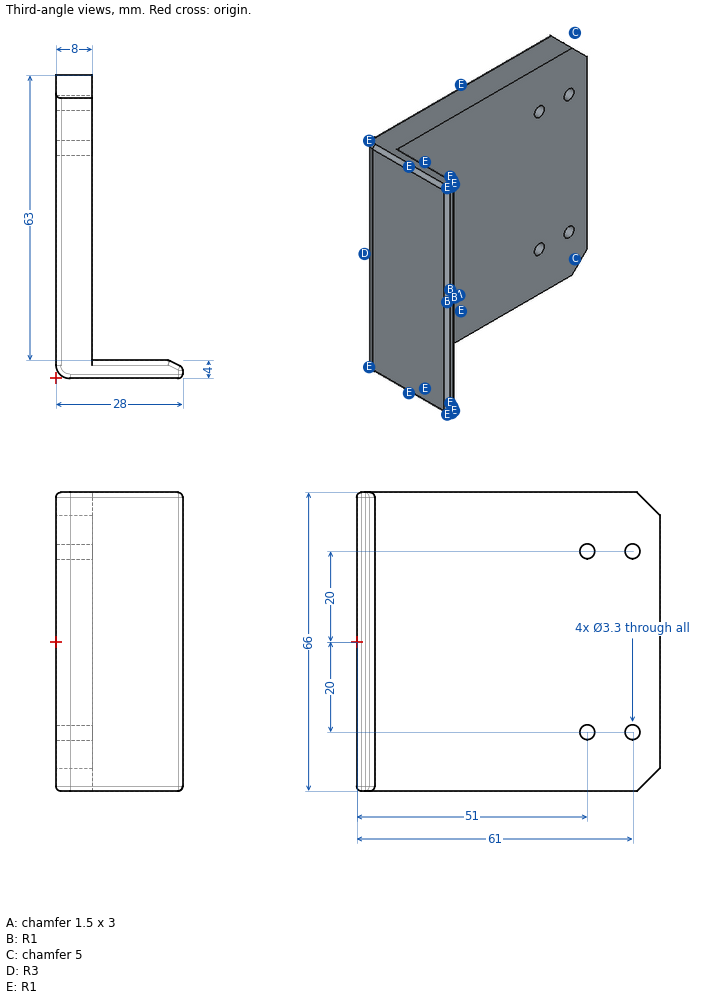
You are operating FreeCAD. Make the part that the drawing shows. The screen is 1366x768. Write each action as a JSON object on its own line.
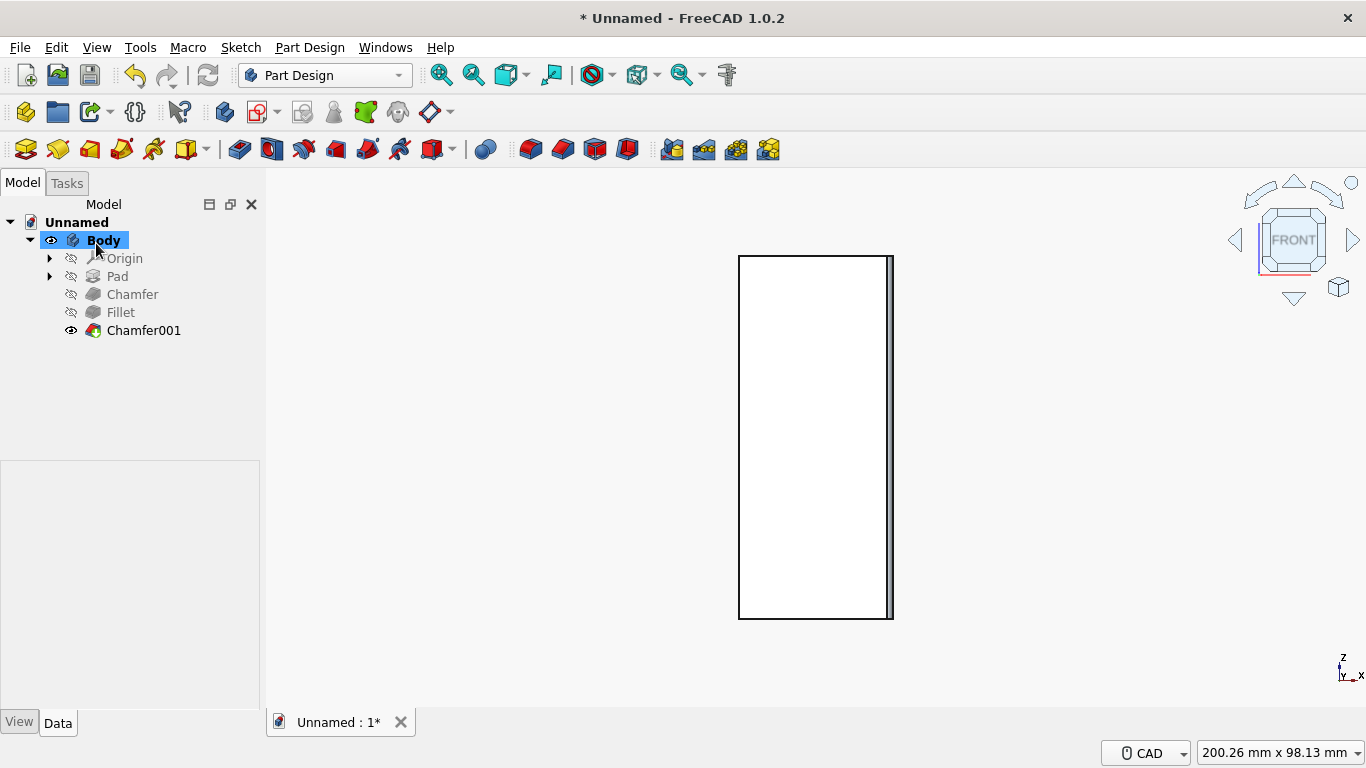
{"action": "left_click", "coordinate": [739, 437]}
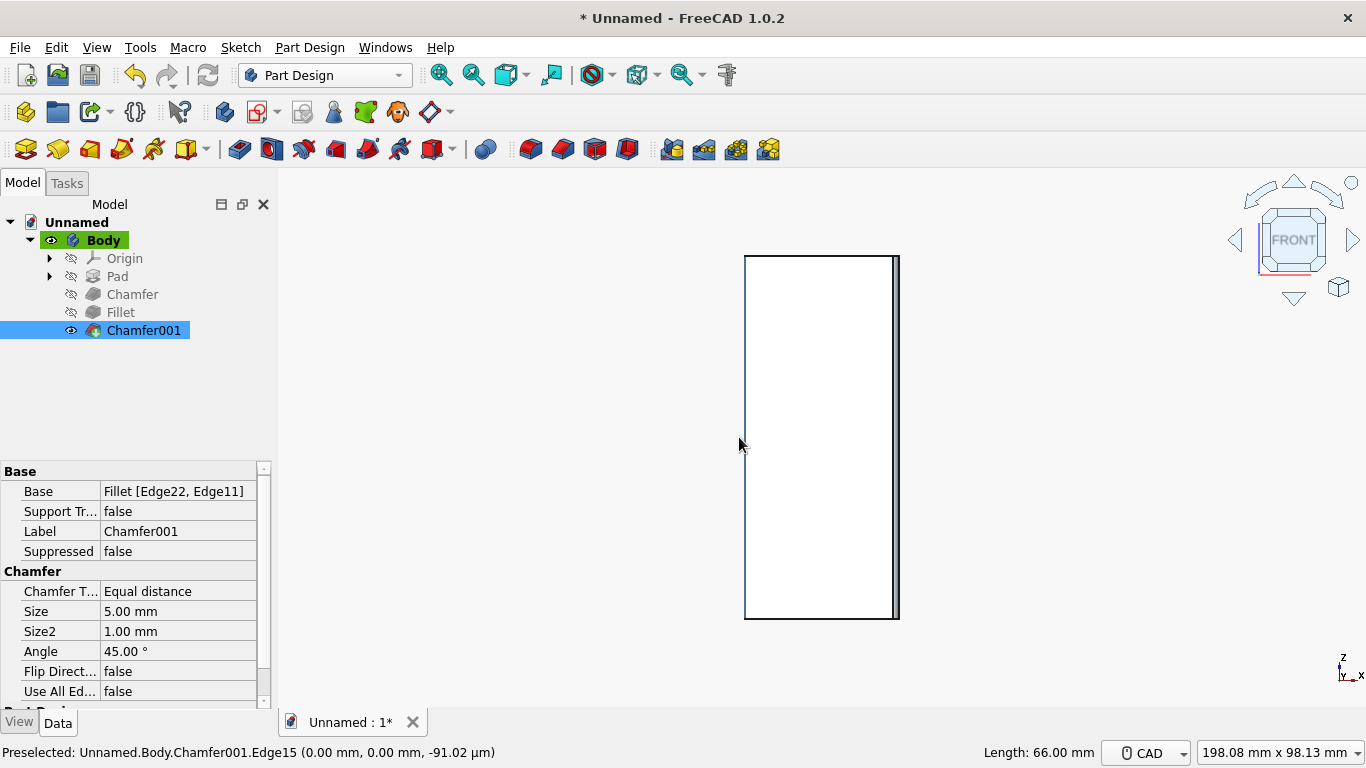
{"action": "left_click", "coordinate": [532, 150]}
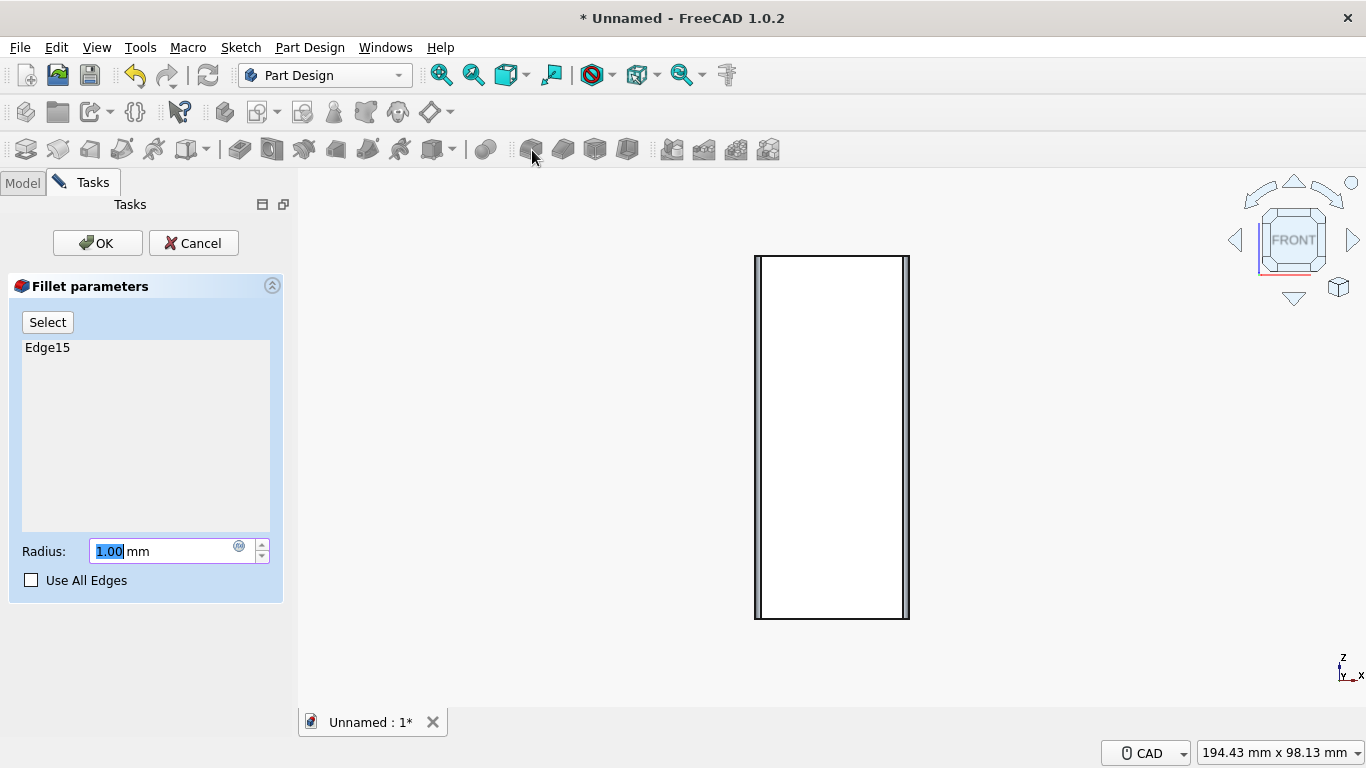
{"action": "type", "text": "3"}
{"action": "key", "text": "Tab"}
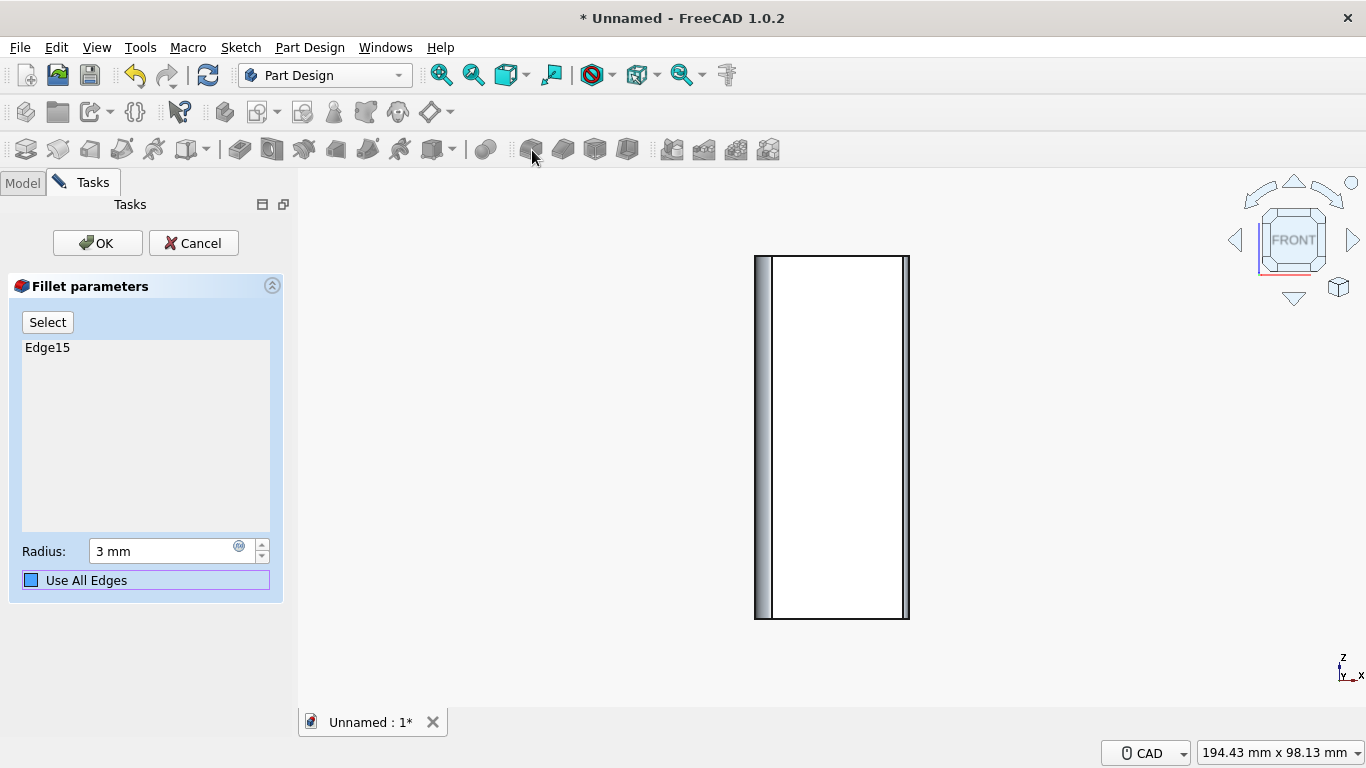
{"action": "left_click", "coordinate": [98, 243]}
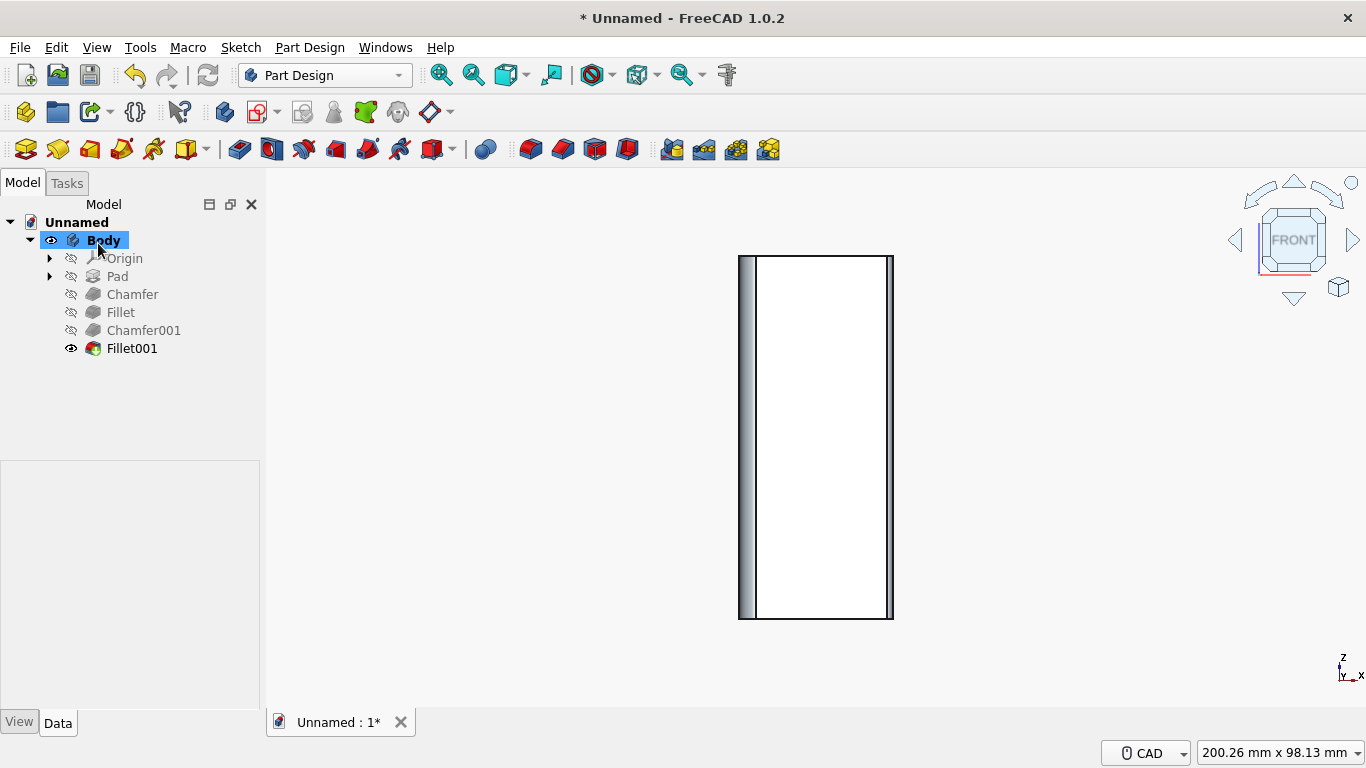
{"action": "left_click", "coordinate": [821, 618]}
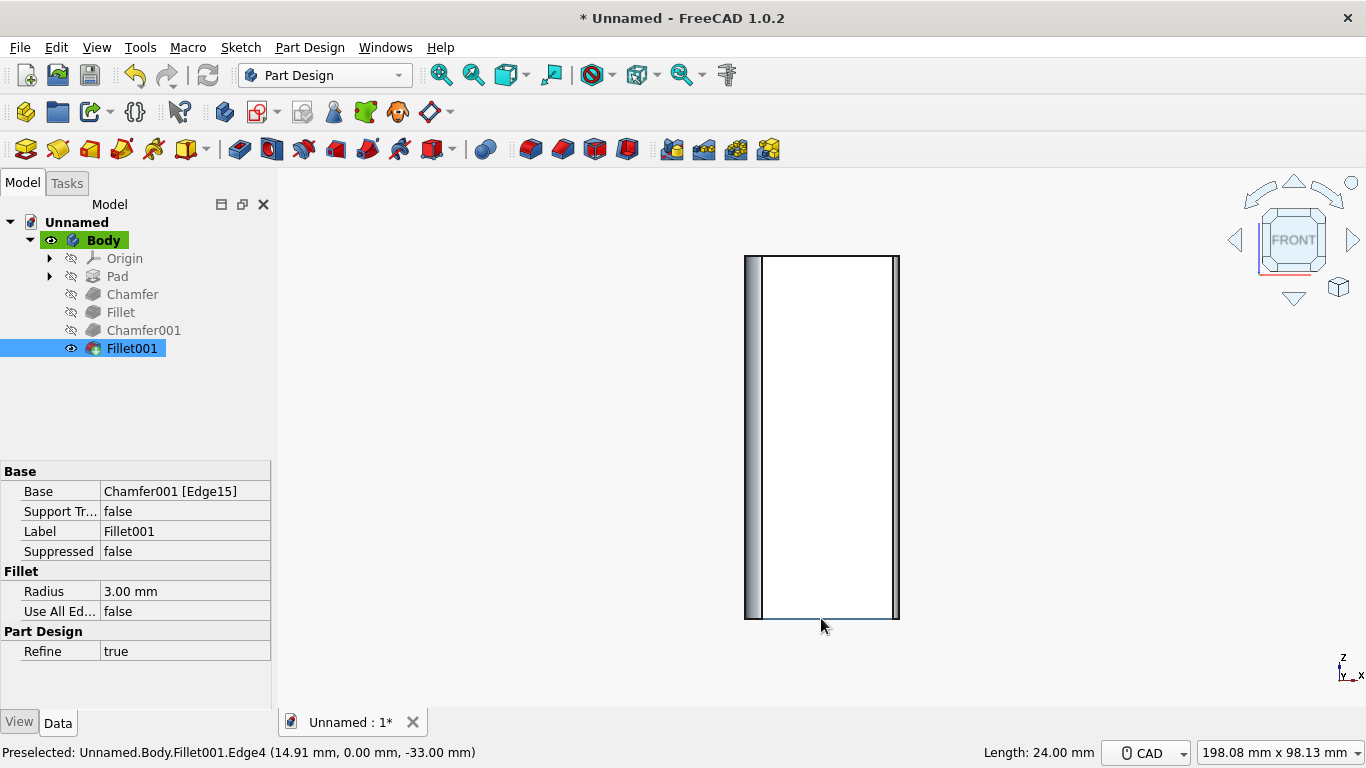
{"action": "left_click", "coordinate": [827, 255], "text": "ctrl"}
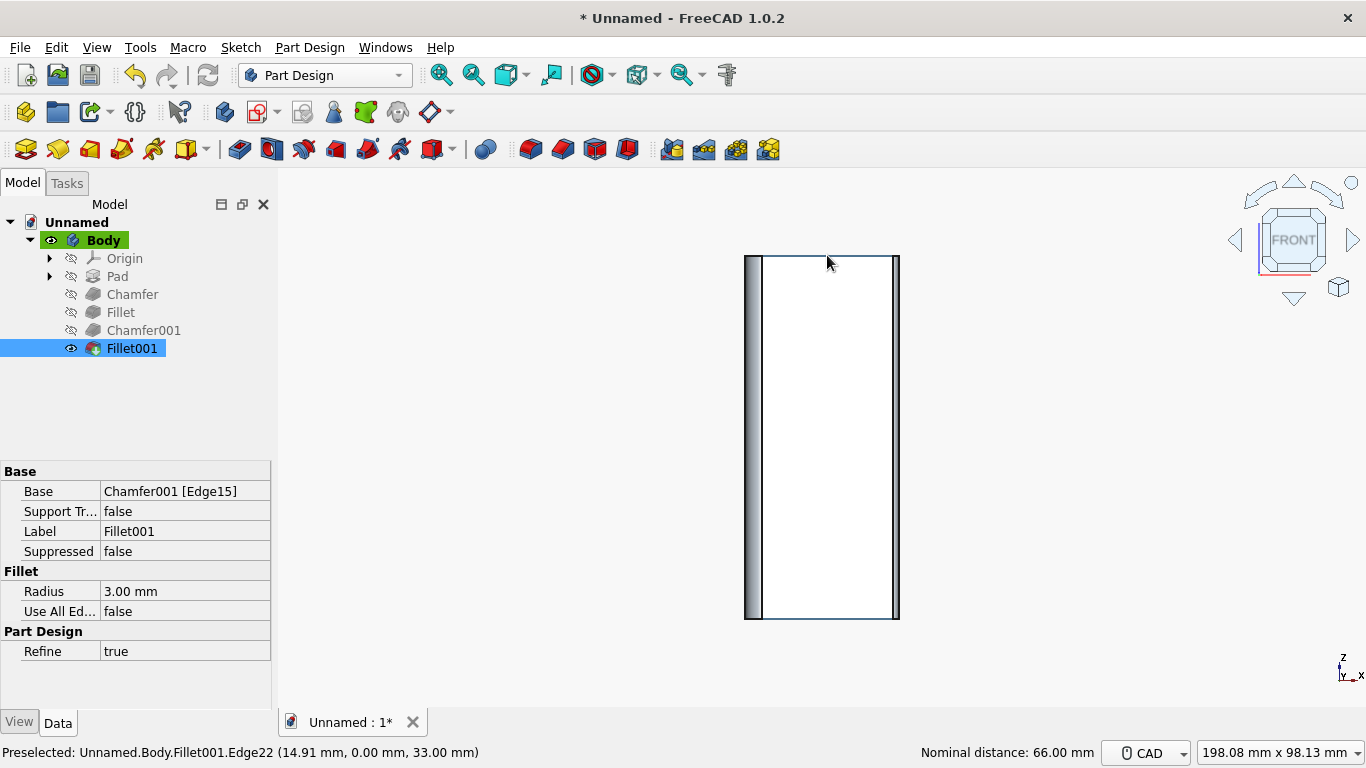
{"action": "left_click", "coordinate": [750, 618], "text": "ctrl"}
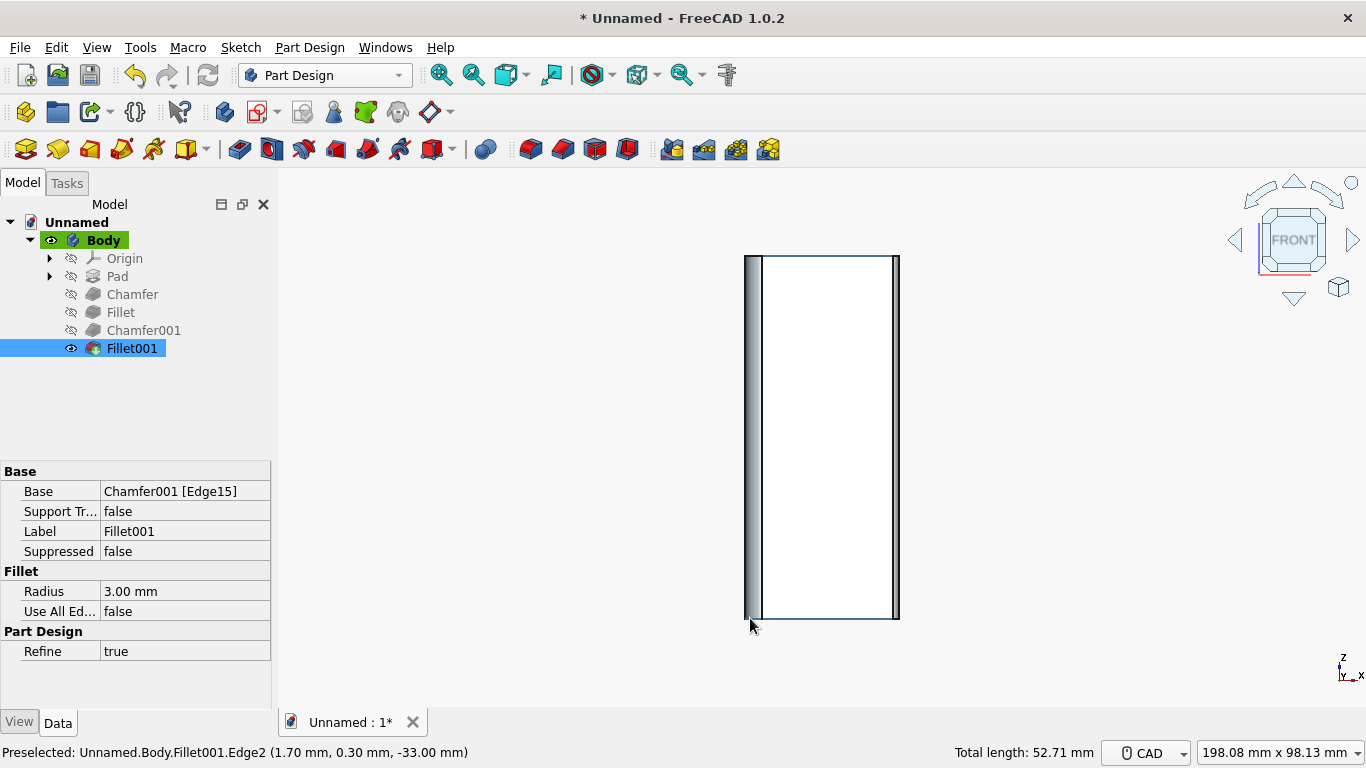
{"action": "left_click", "coordinate": [750, 255], "text": "ctrl"}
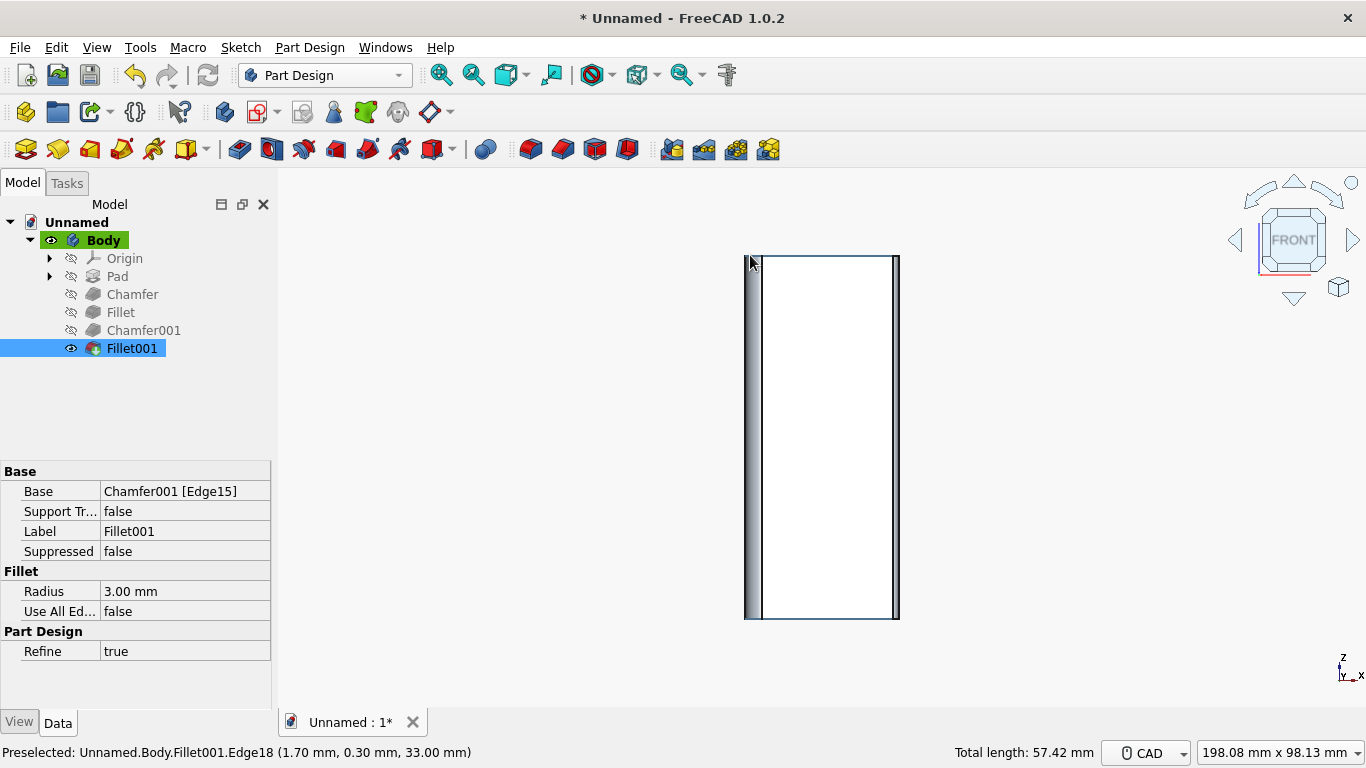
{"action": "scroll", "coordinate": [899, 618], "scroll_direction": "up", "scroll_amount": 11}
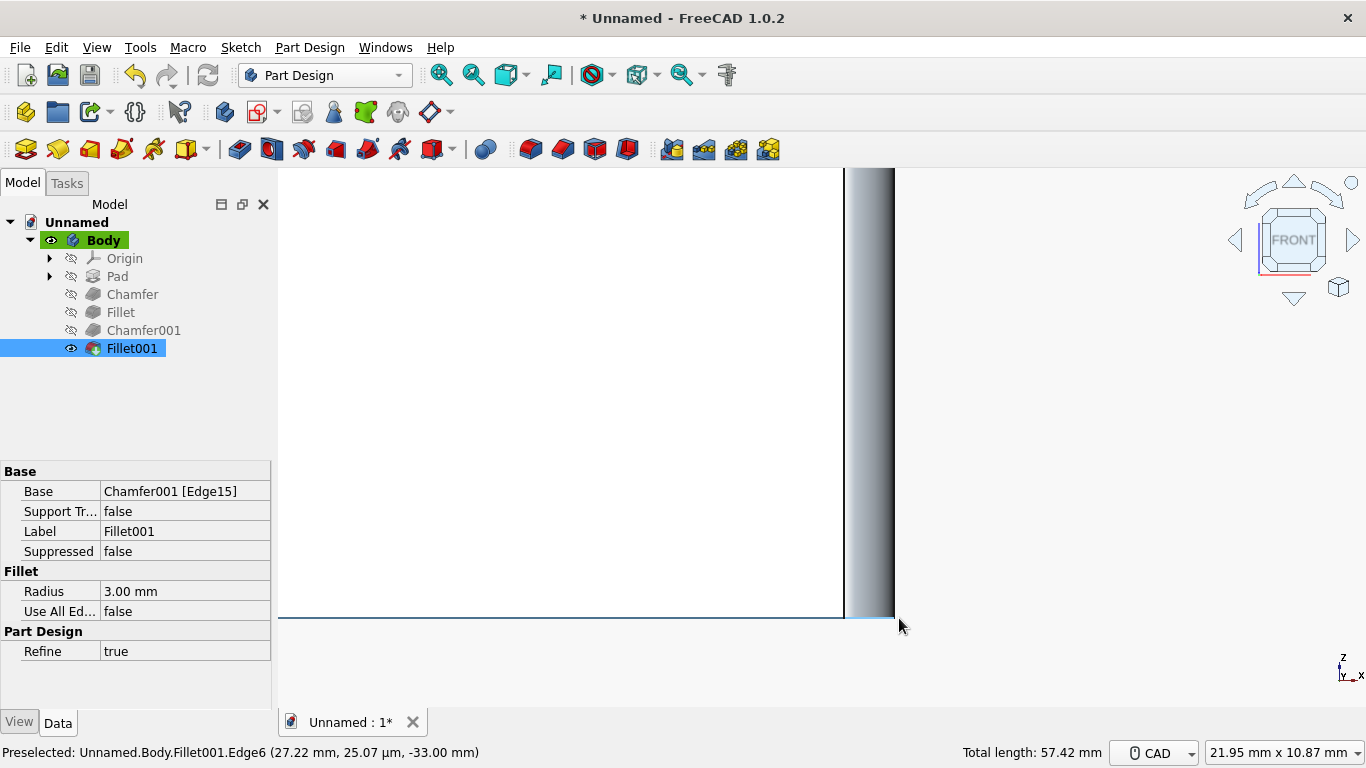
{"action": "left_click", "coordinate": [879, 617], "text": "ctrl"}